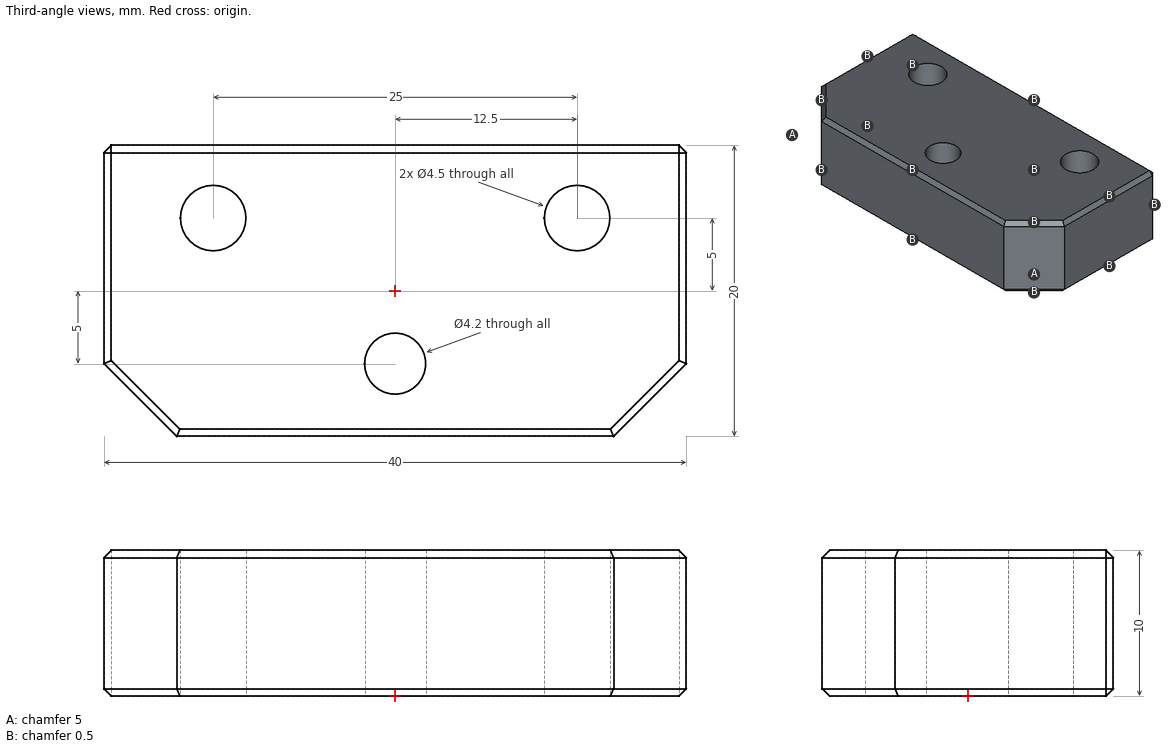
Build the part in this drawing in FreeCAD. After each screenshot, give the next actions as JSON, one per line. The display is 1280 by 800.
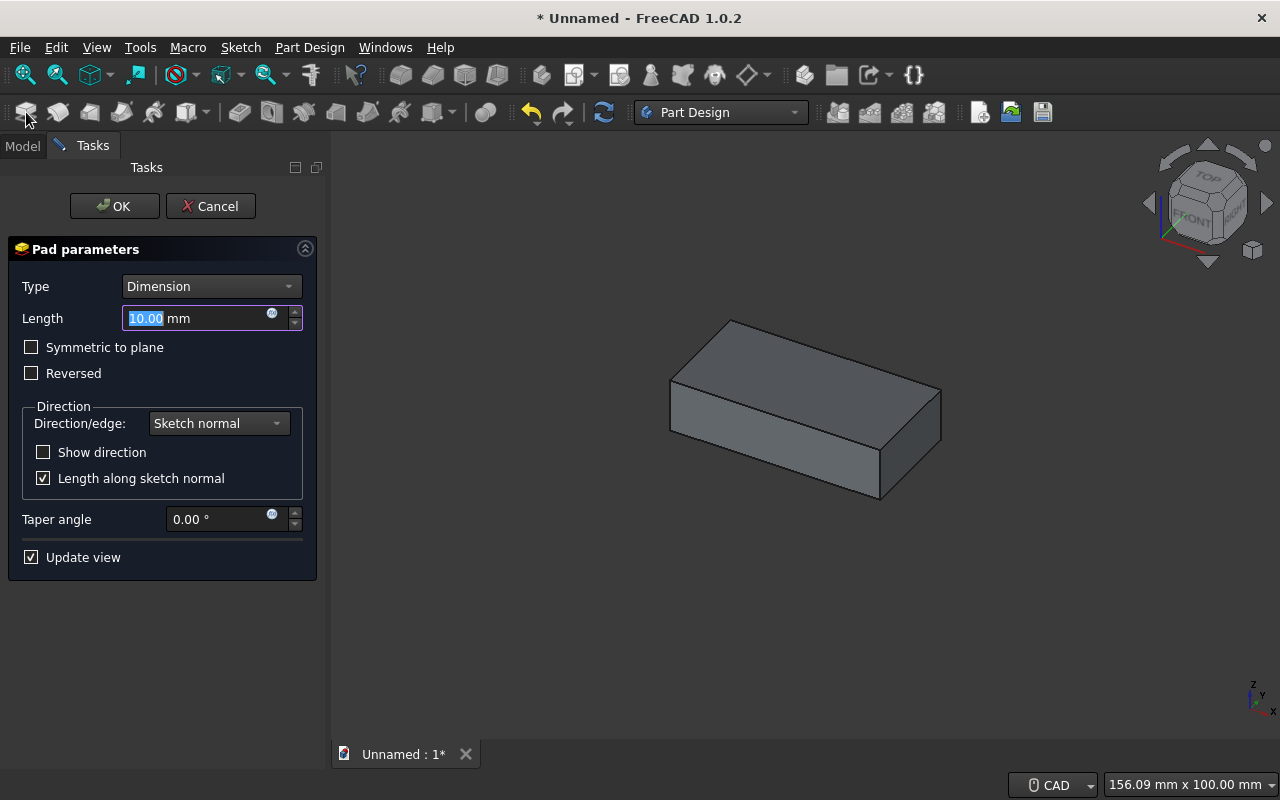
{"action": "type", "text": "10"}
{"action": "key", "text": "Tab"}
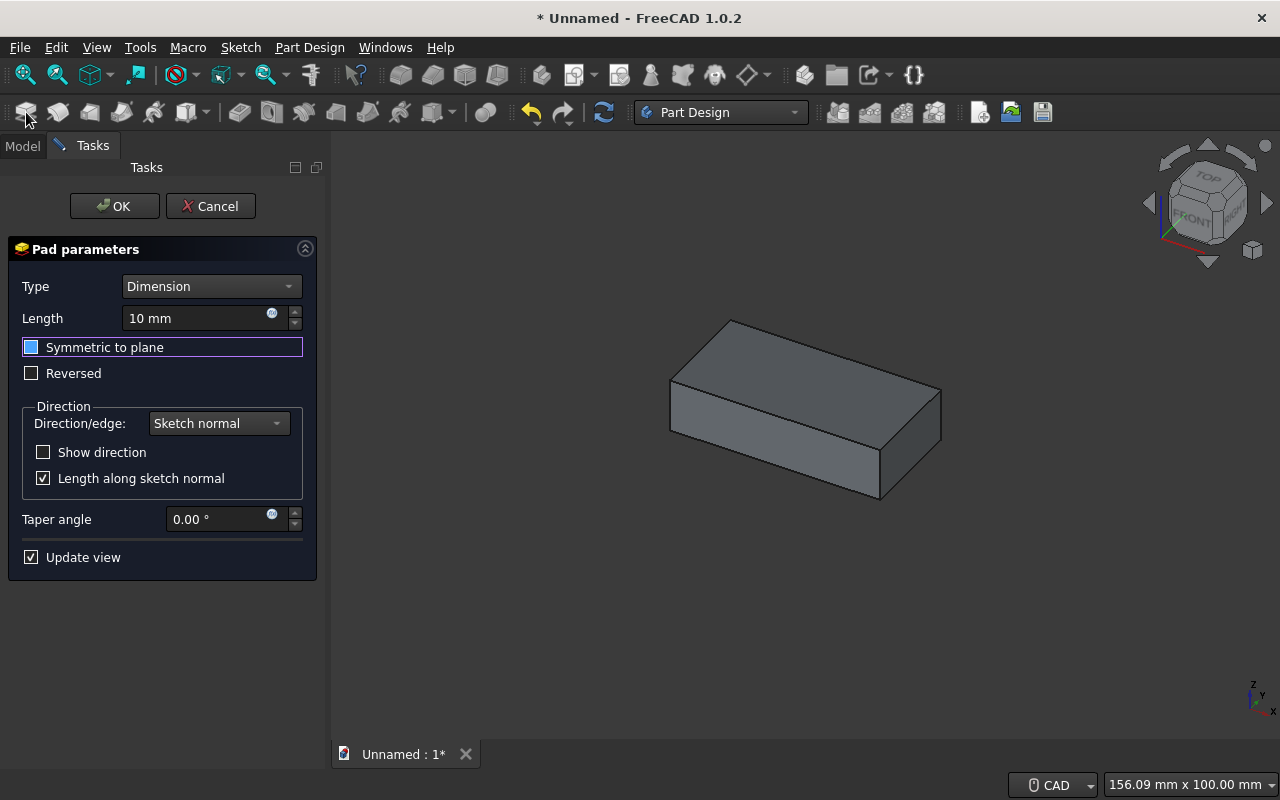
{"action": "left_click", "coordinate": [115, 206]}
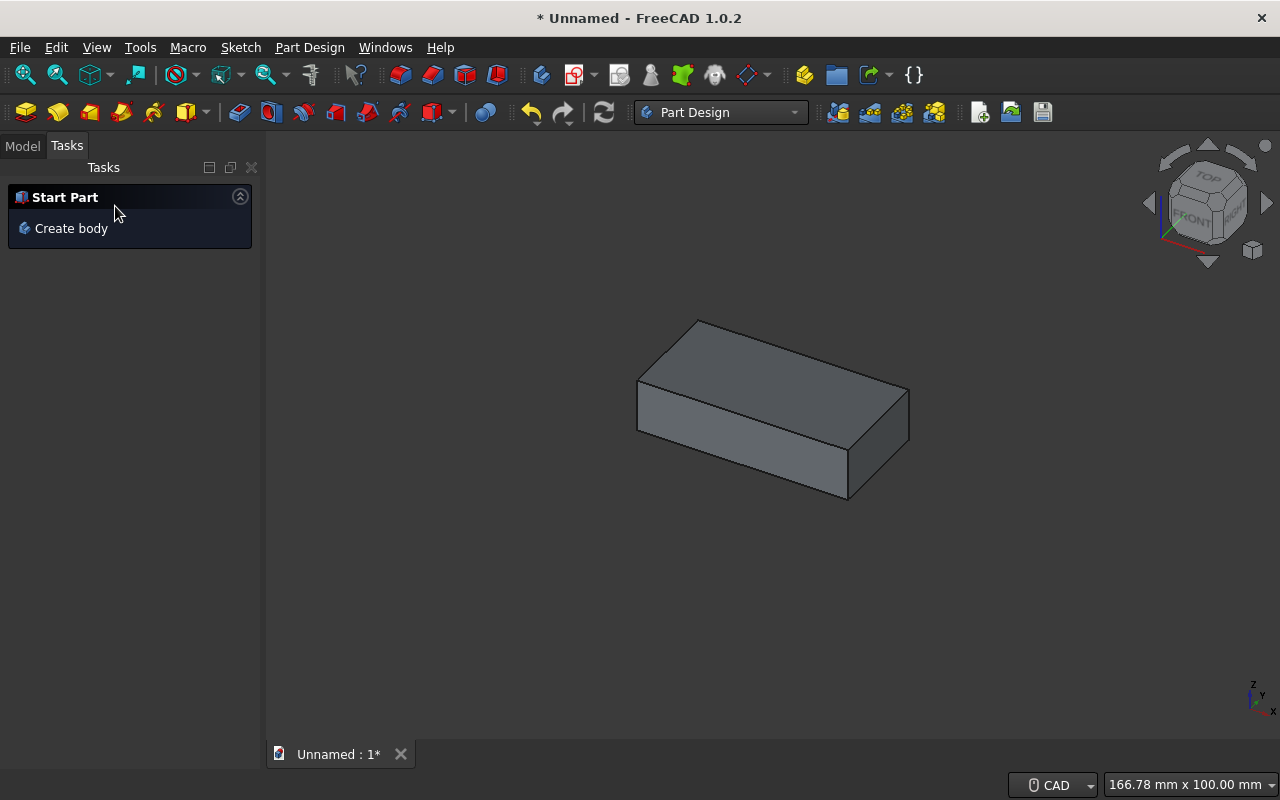
{"action": "left_click", "coordinate": [26, 76]}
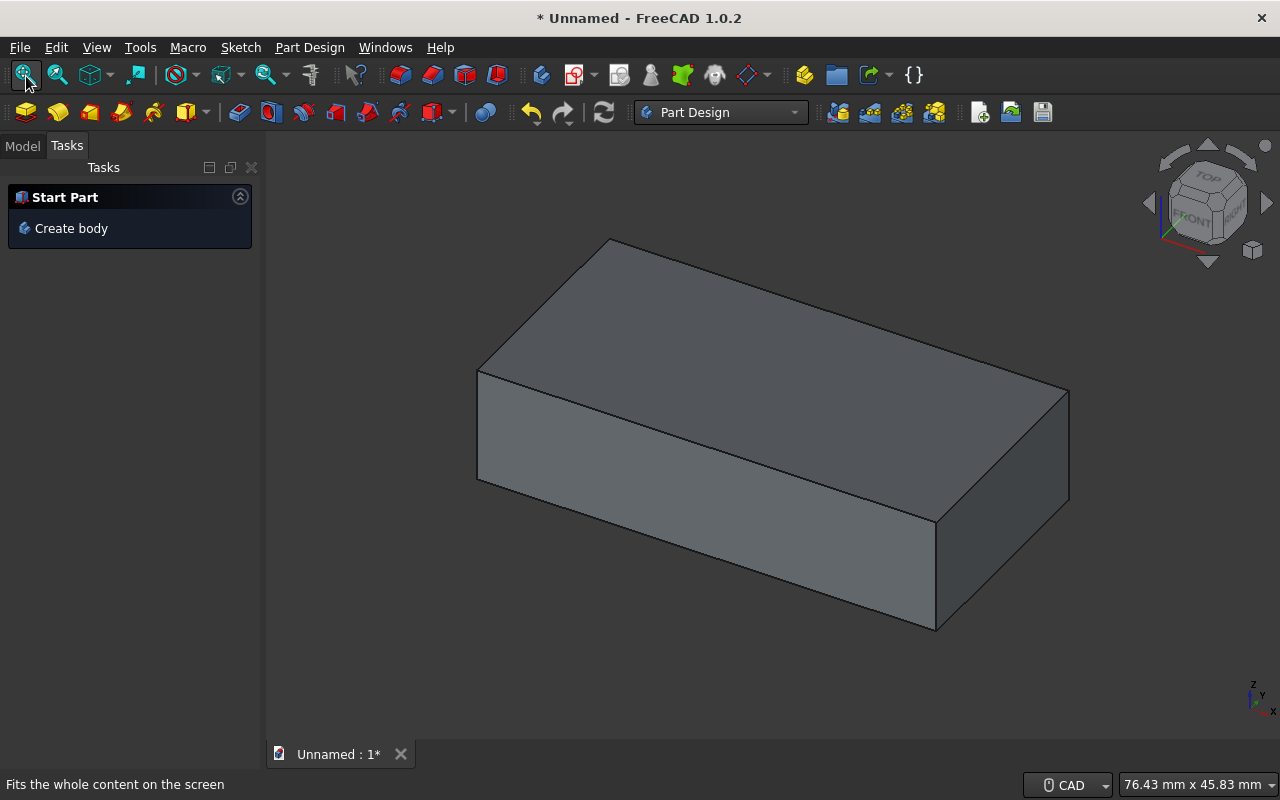
{"action": "left_click", "coordinate": [839, 401]}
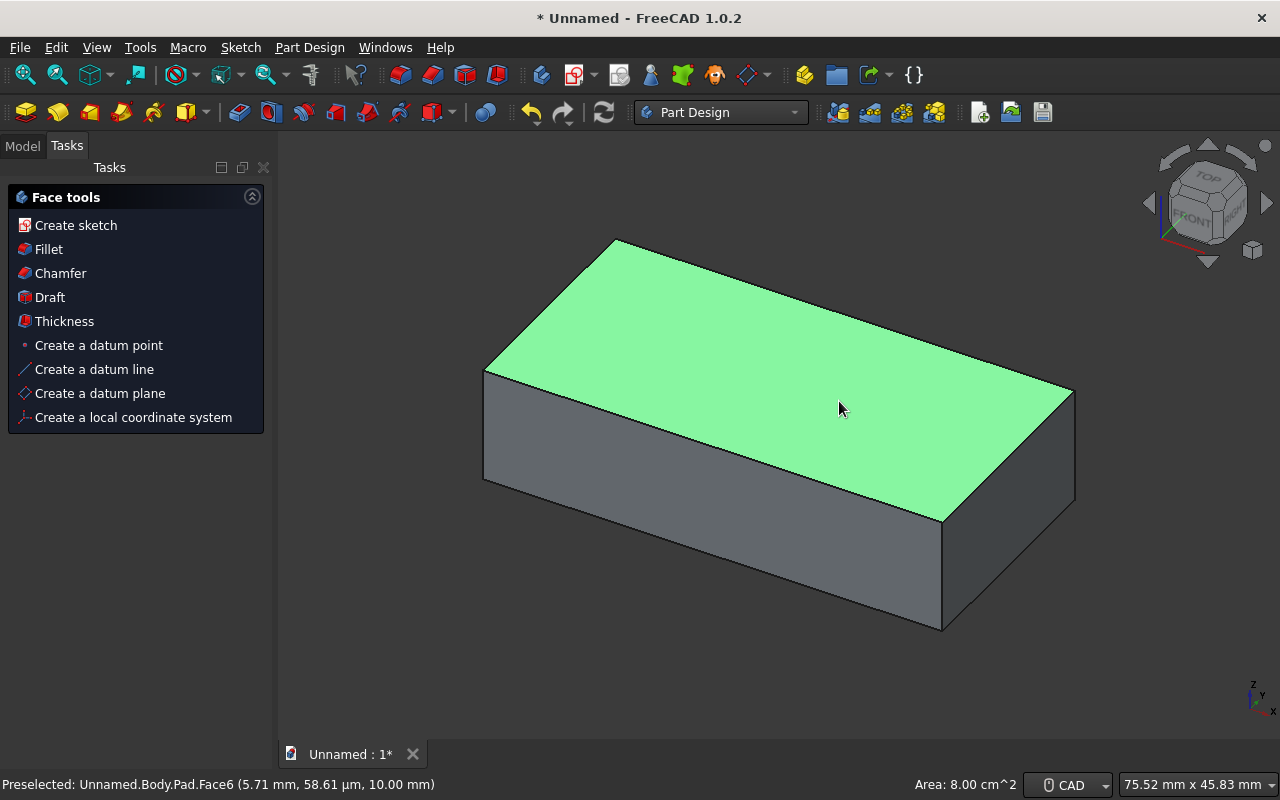
{"action": "left_click", "coordinate": [574, 76]}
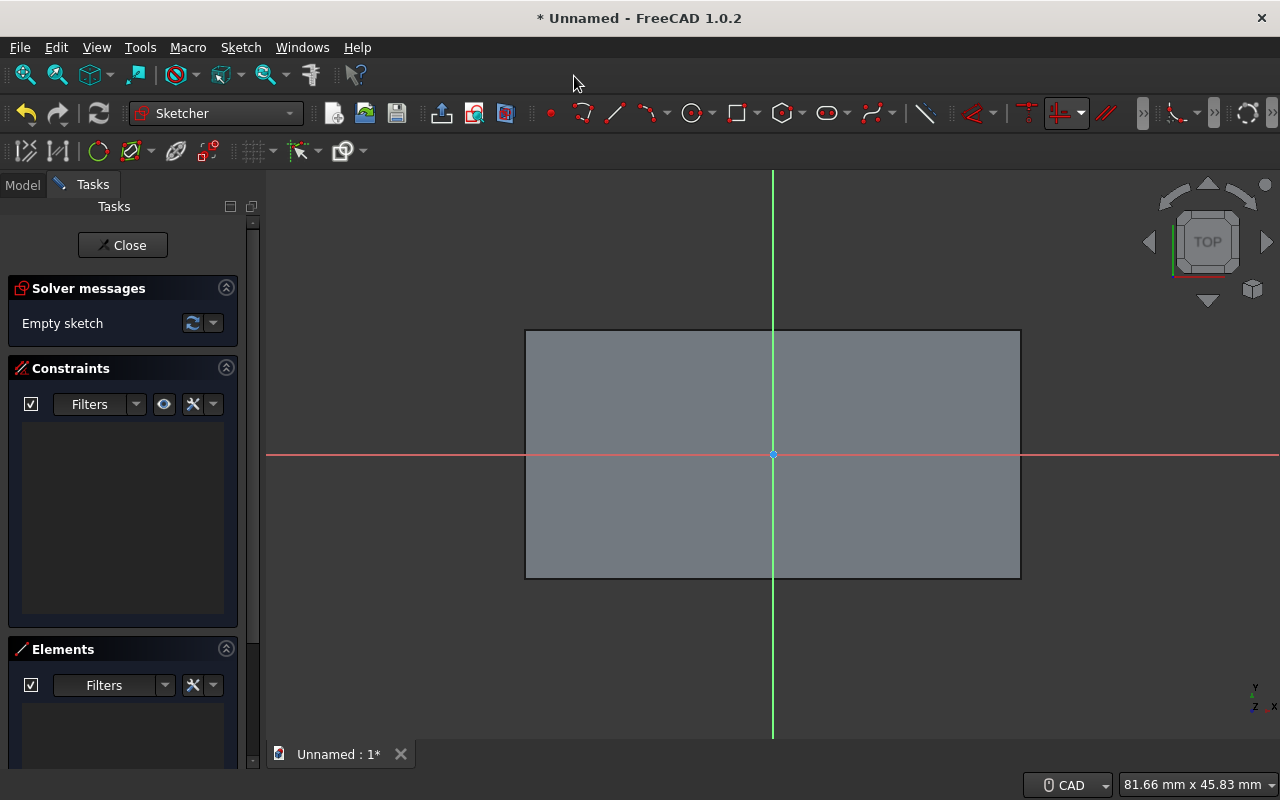
{"action": "scroll", "coordinate": [912, 318], "scroll_direction": "up", "scroll_amount": 2}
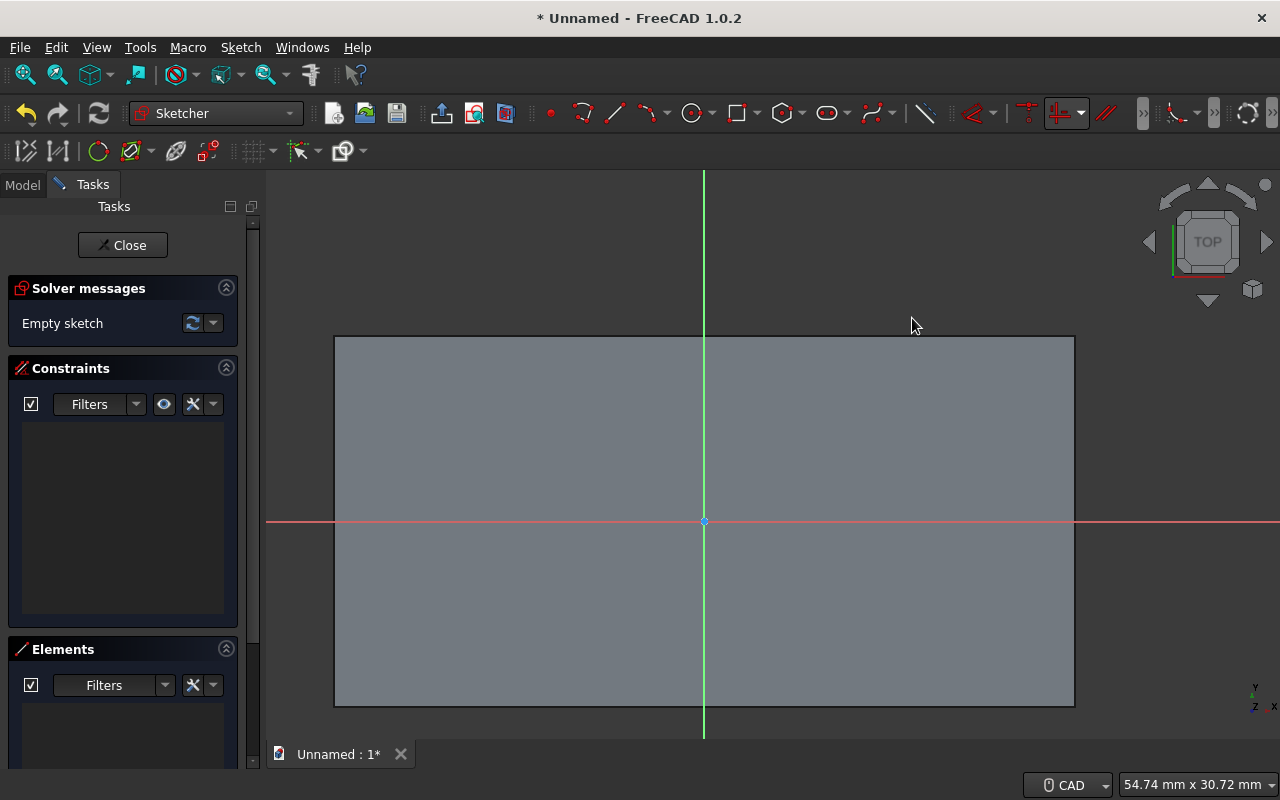
{"action": "left_click", "coordinate": [692, 114]}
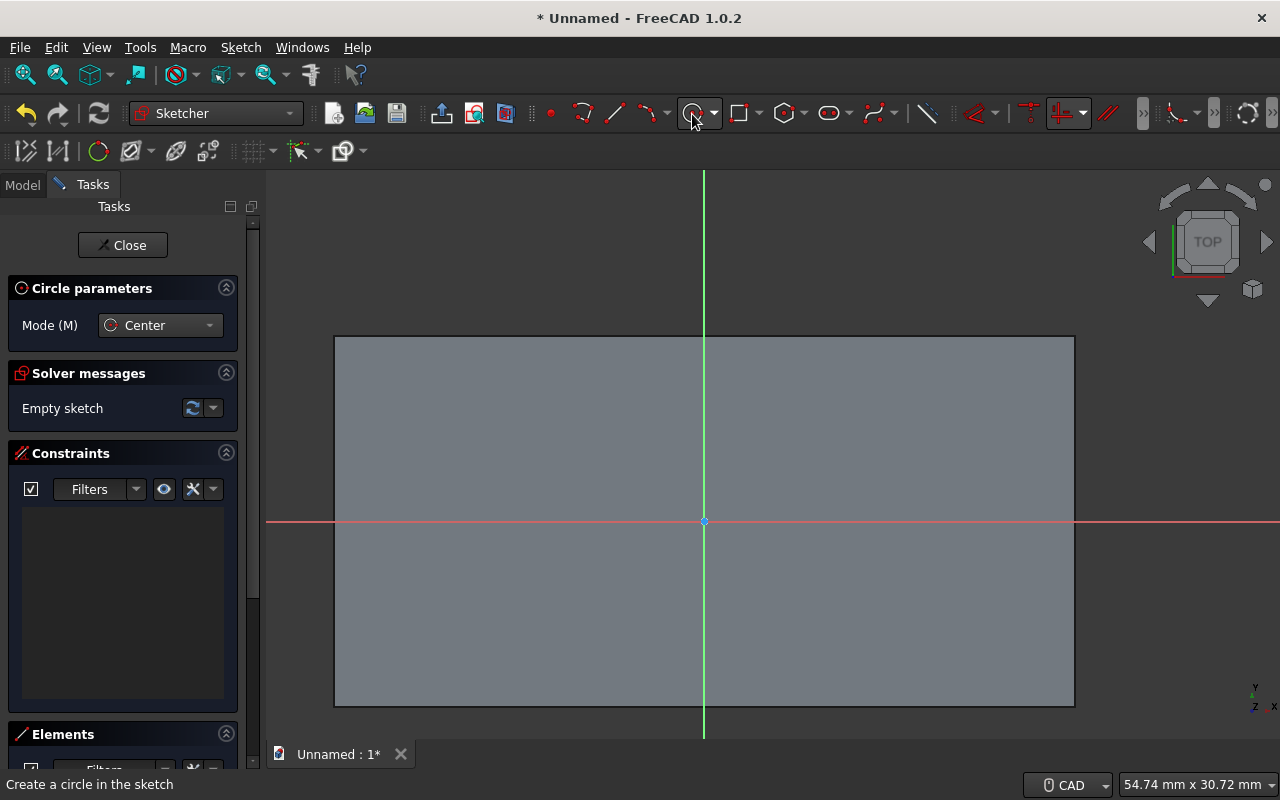
{"action": "left_click", "coordinate": [936, 429]}
{"action": "mouse_move", "coordinate": [965, 399]}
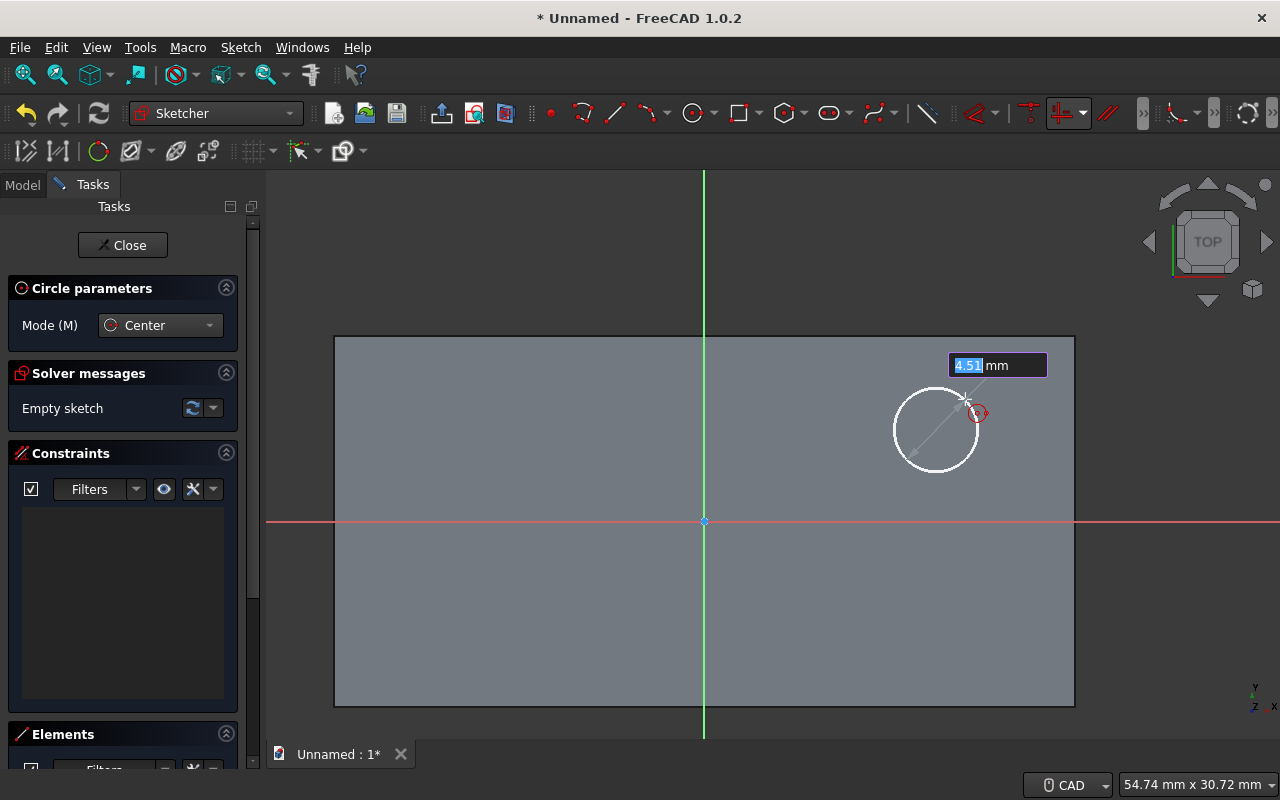
{"action": "type", "text": "4.5"}
{"action": "key", "text": "Return"}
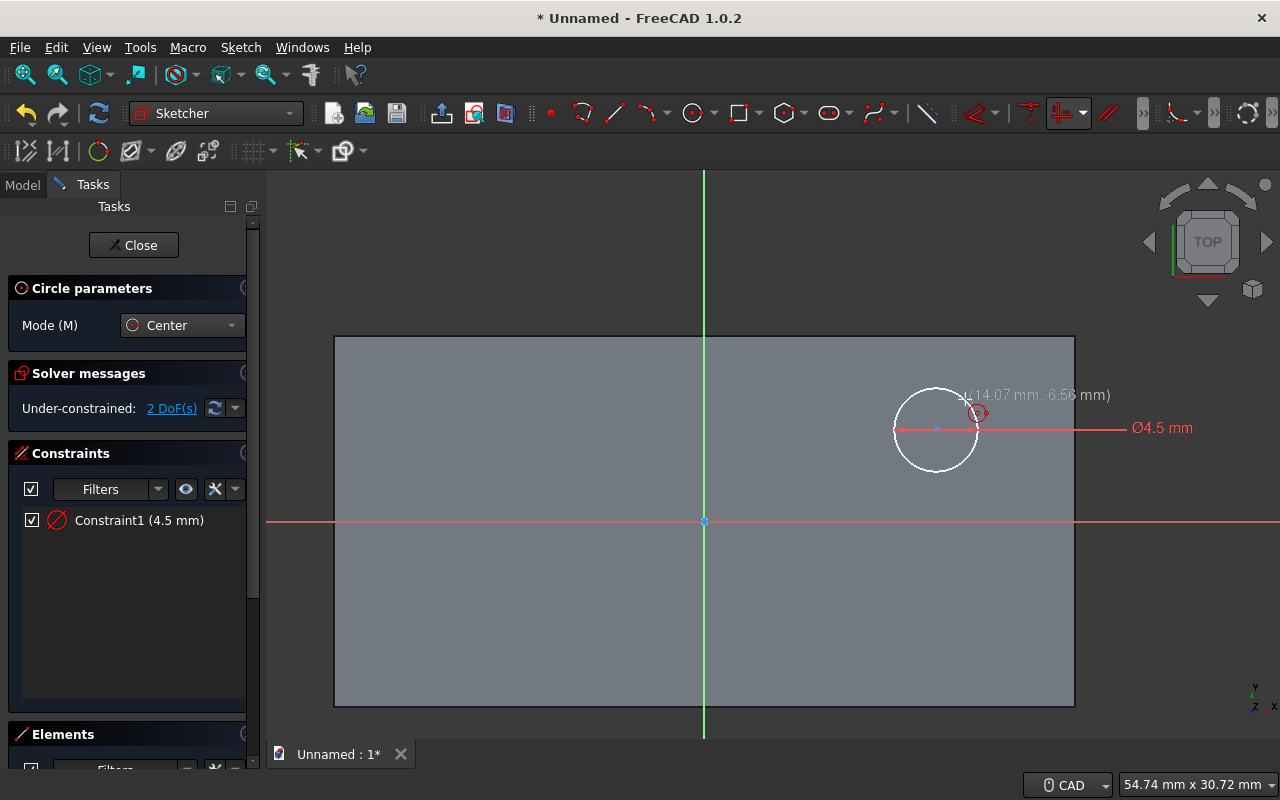
{"action": "left_click", "coordinate": [473, 429]}
{"action": "mouse_move", "coordinate": [502, 399]}